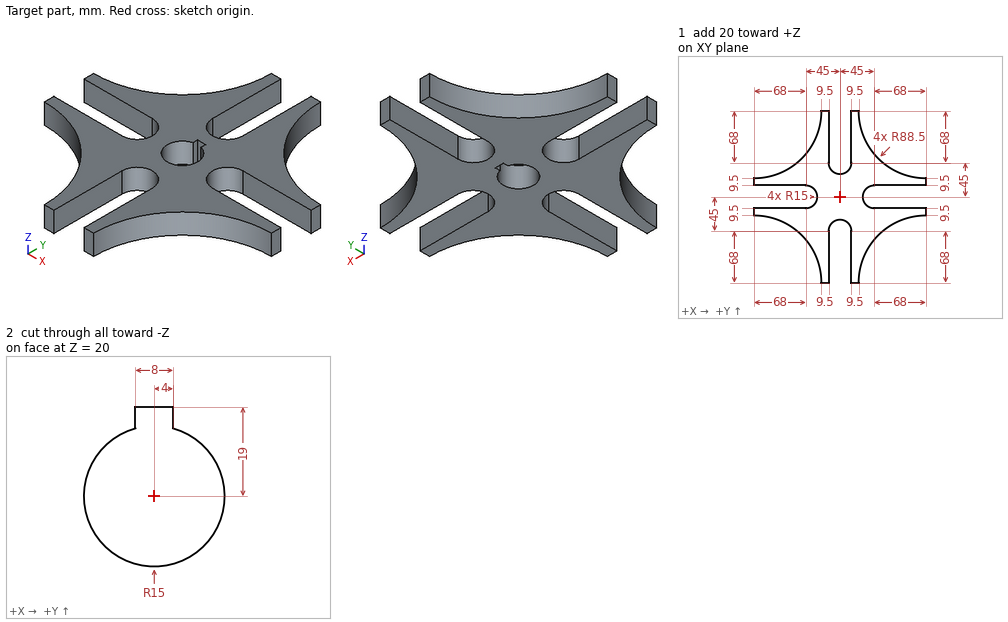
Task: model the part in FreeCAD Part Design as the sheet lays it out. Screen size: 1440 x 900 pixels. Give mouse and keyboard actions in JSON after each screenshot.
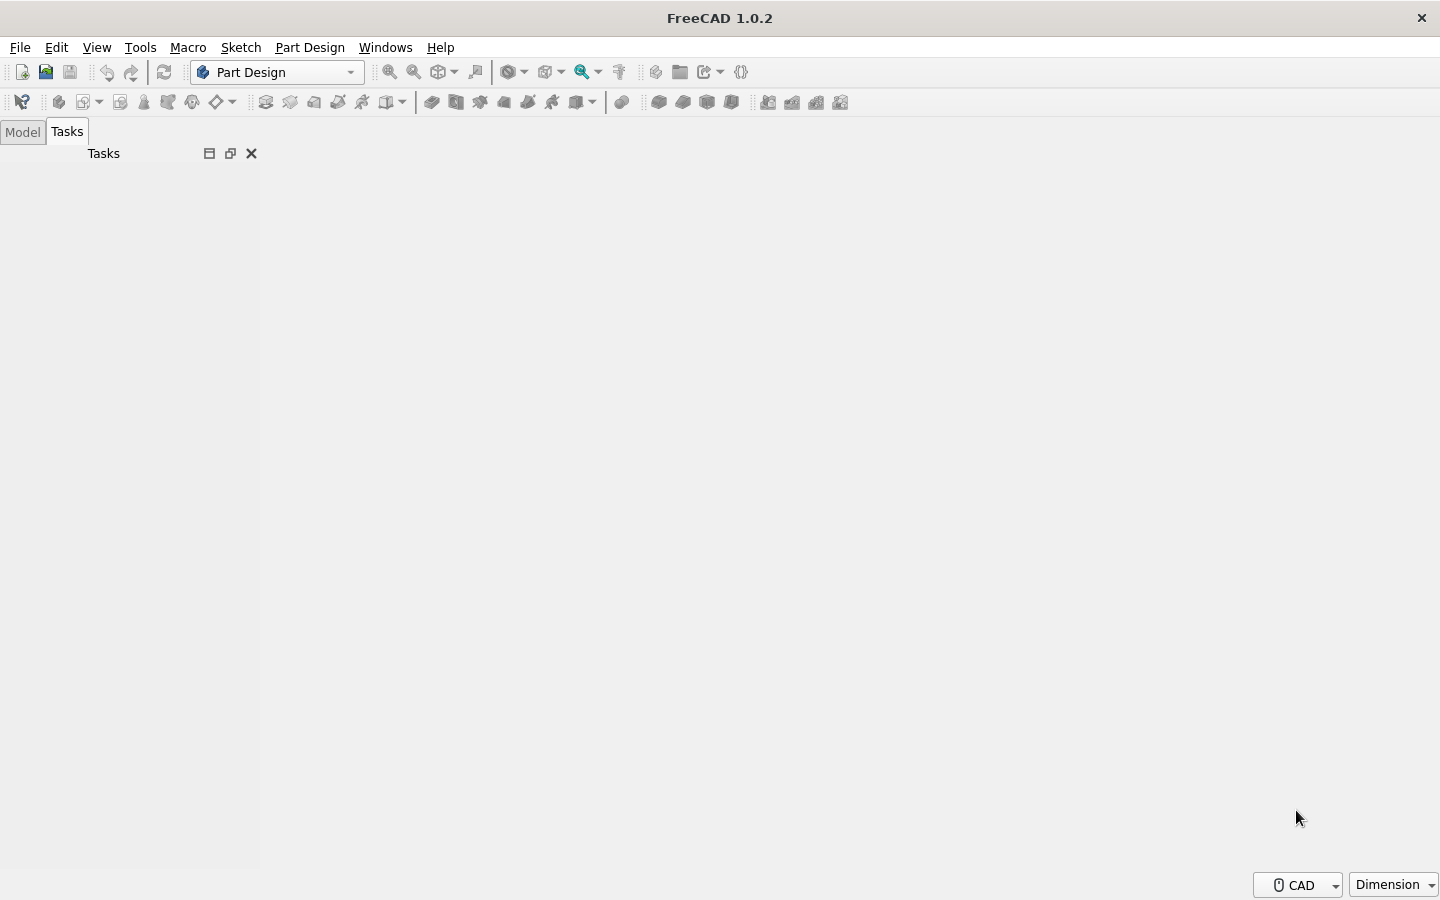
{"action": "left_click", "coordinate": [22, 72]}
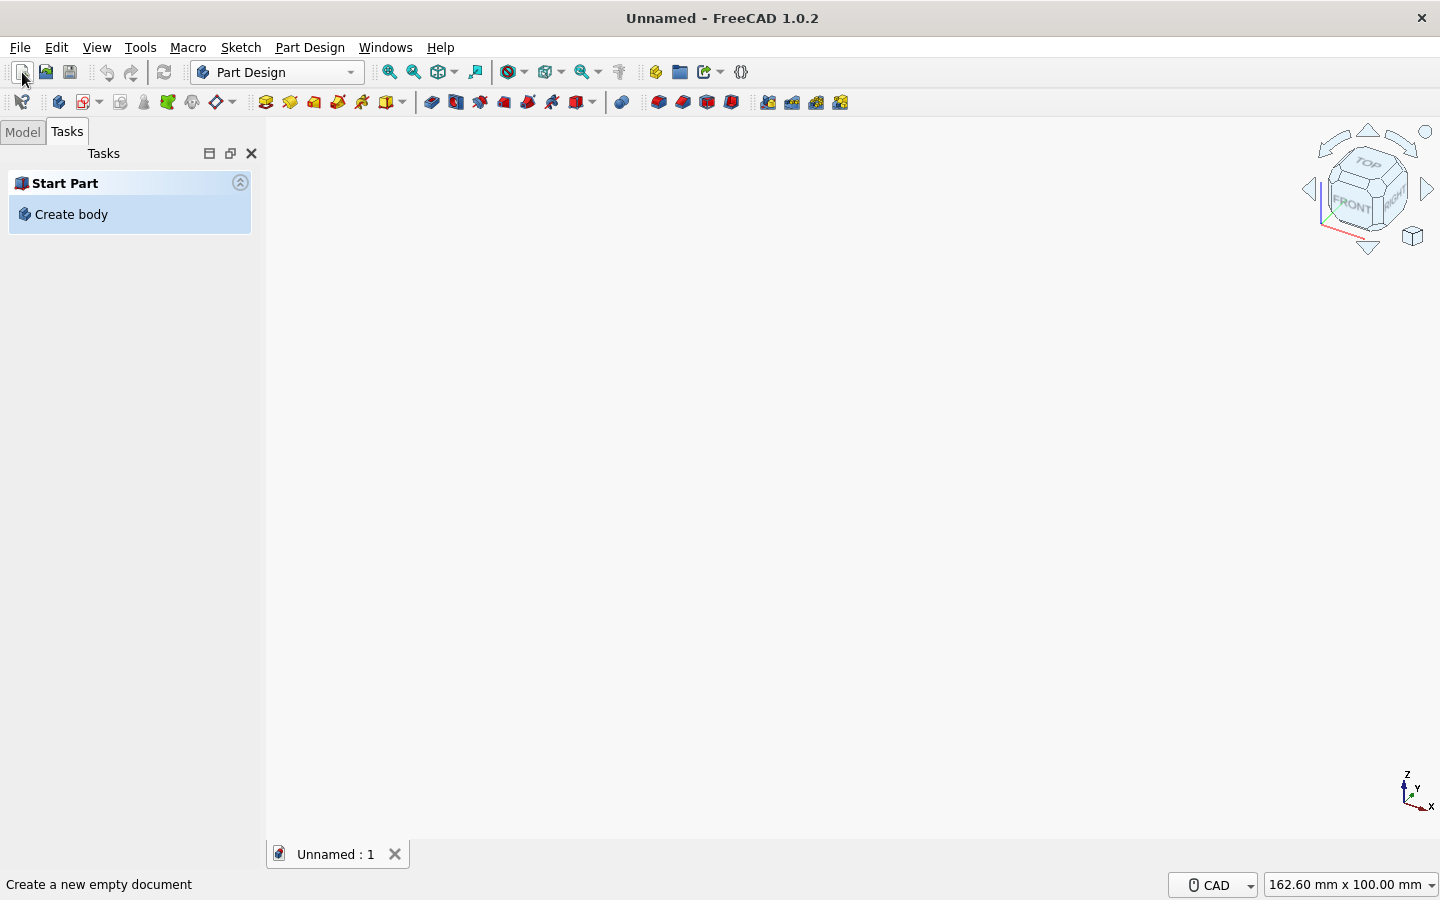
{"action": "left_click", "coordinate": [84, 102]}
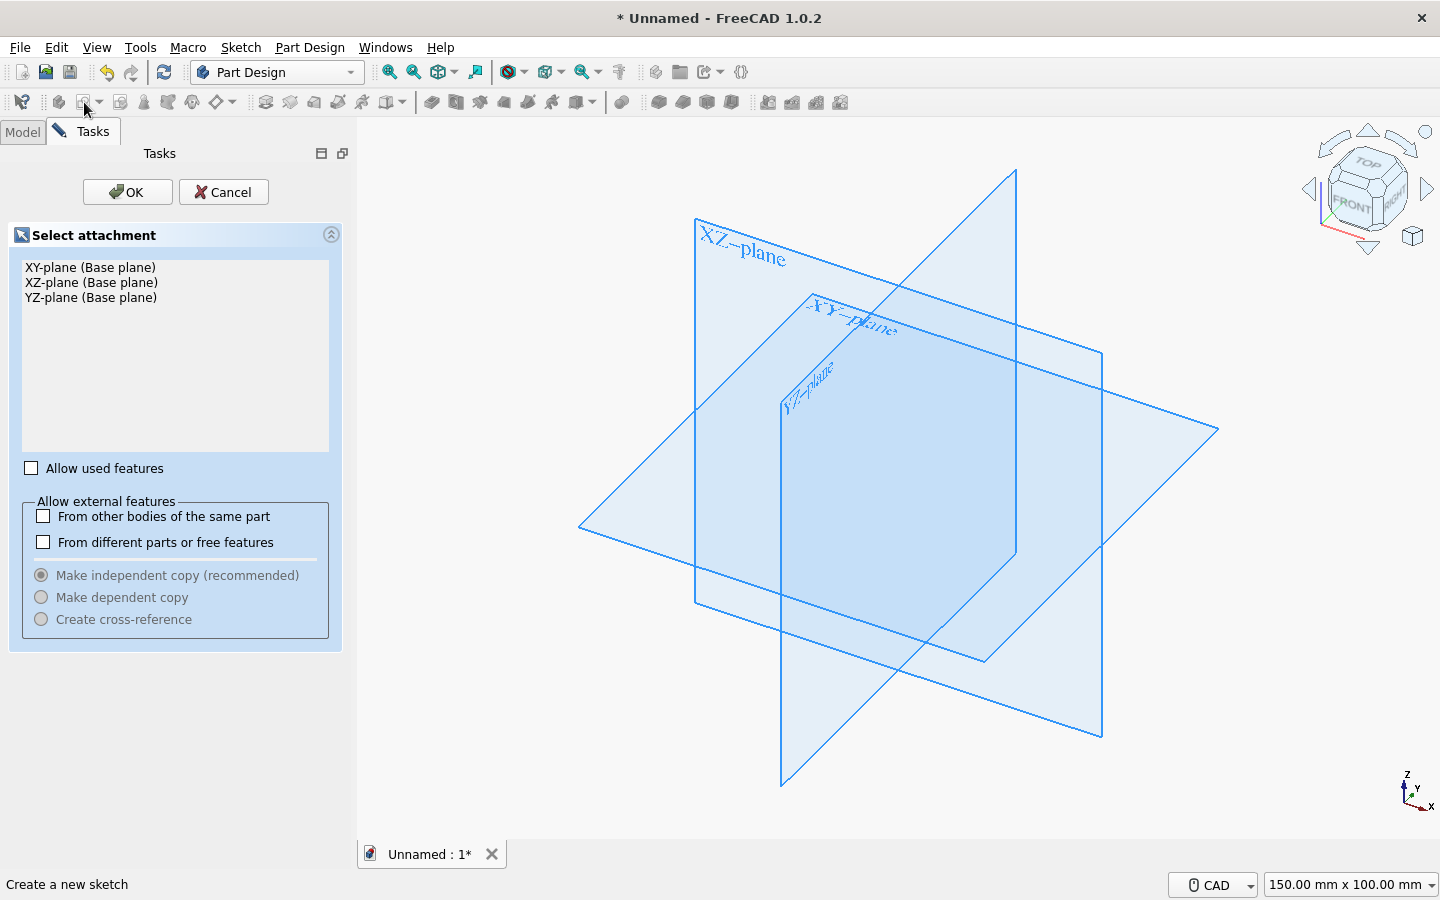
{"action": "left_click", "coordinate": [82, 268]}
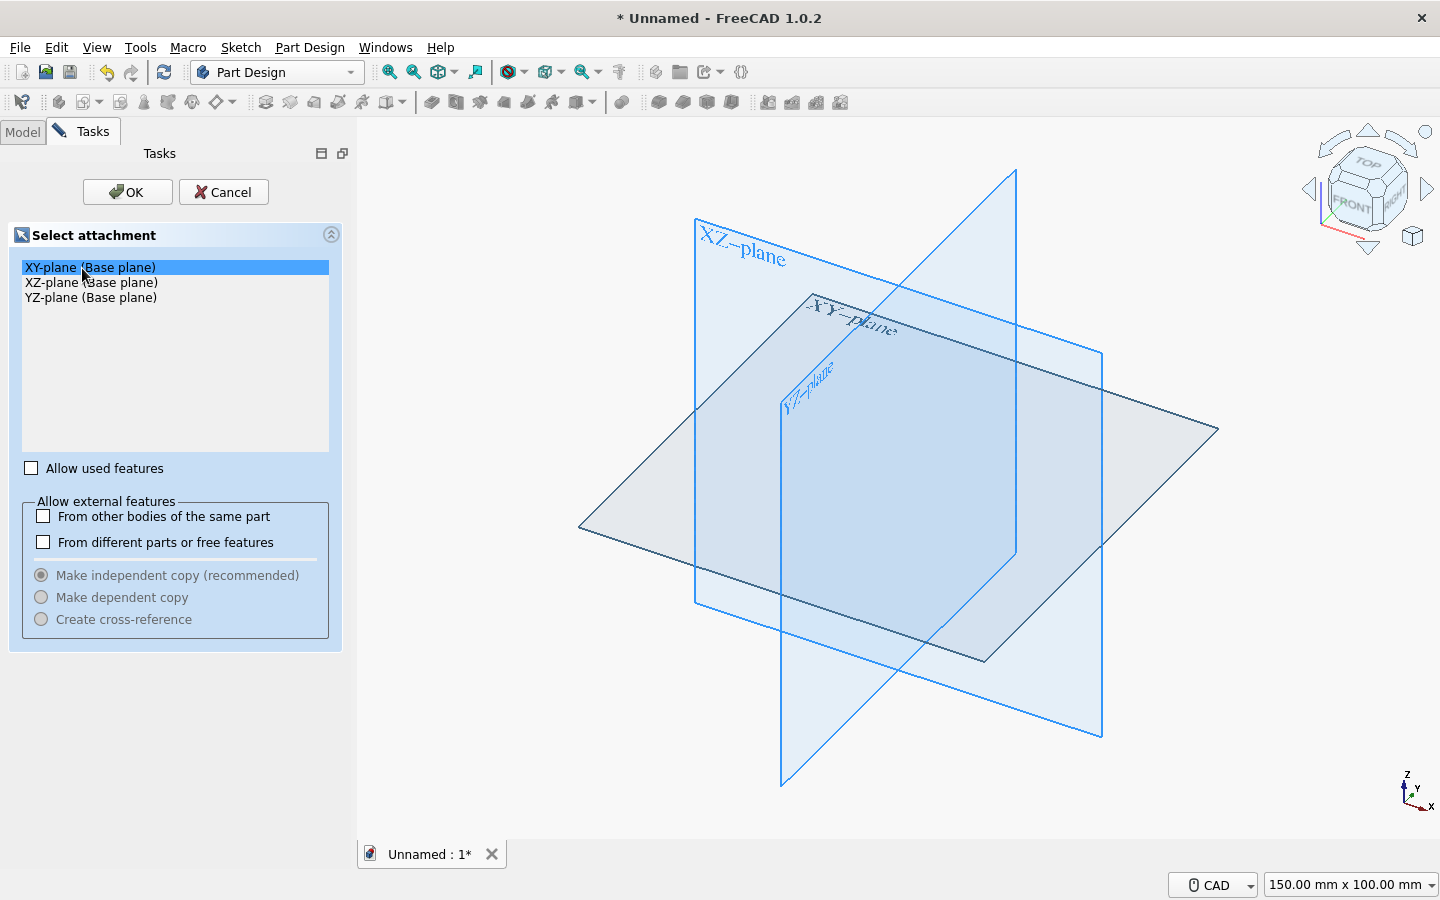
{"action": "left_click", "coordinate": [128, 192]}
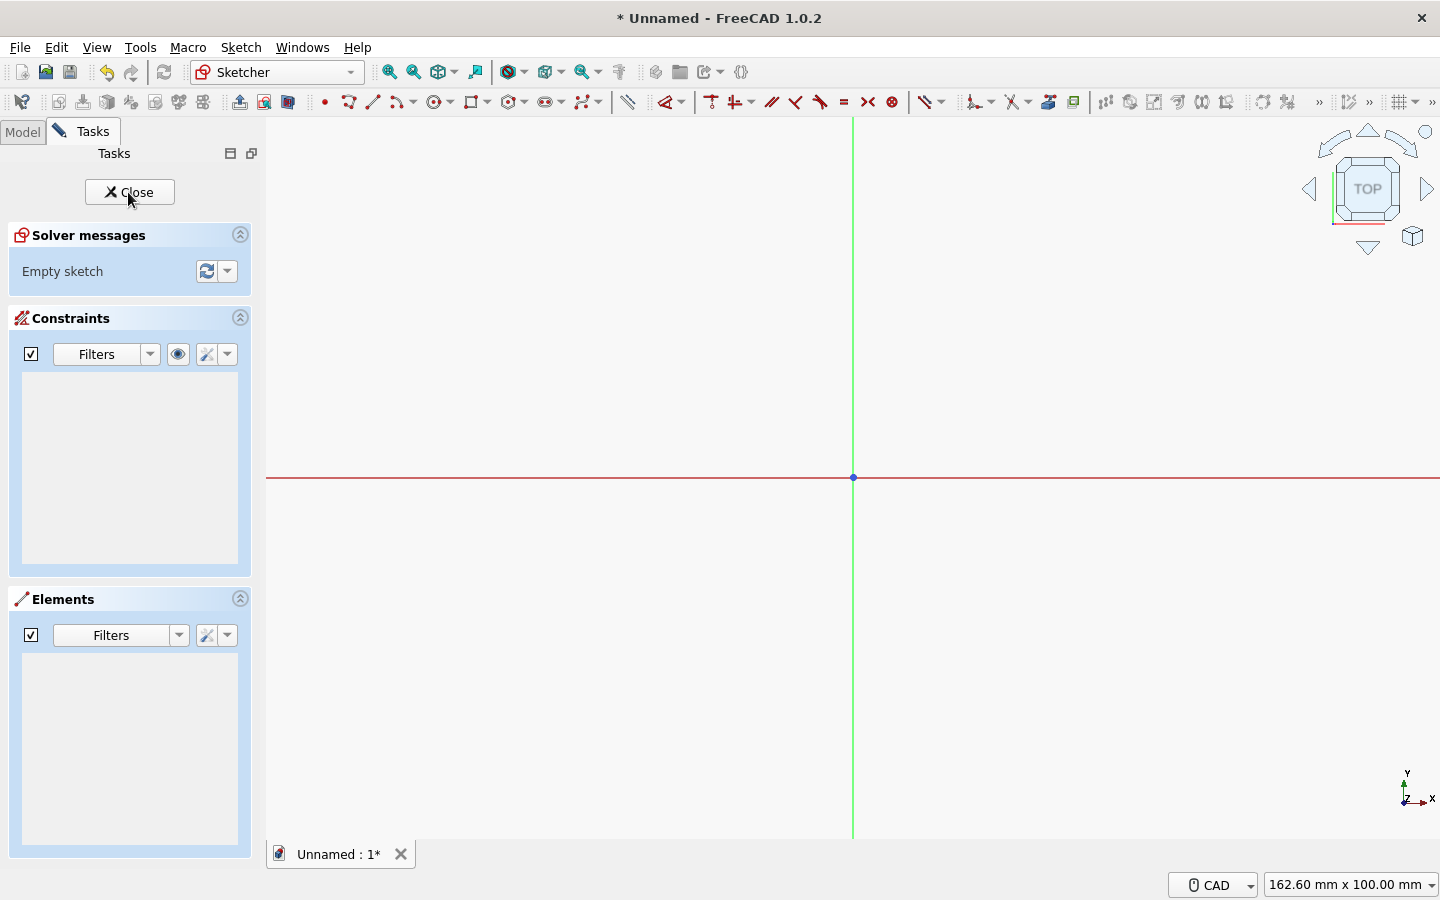
{"action": "scroll", "coordinate": [755, 478], "scroll_direction": "down", "scroll_amount": 6}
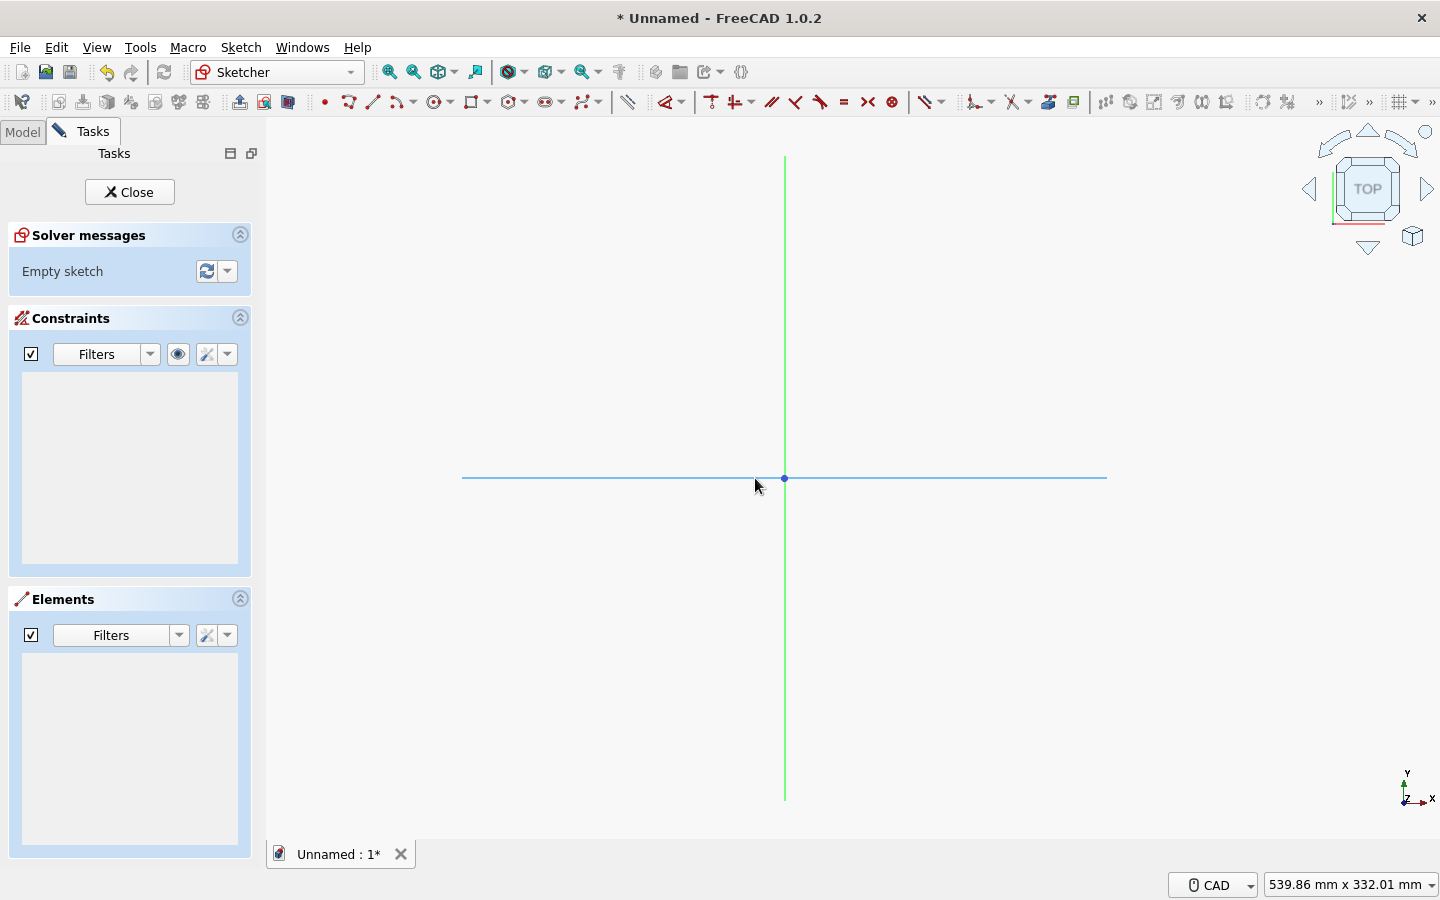
{"action": "left_click", "coordinate": [350, 102]}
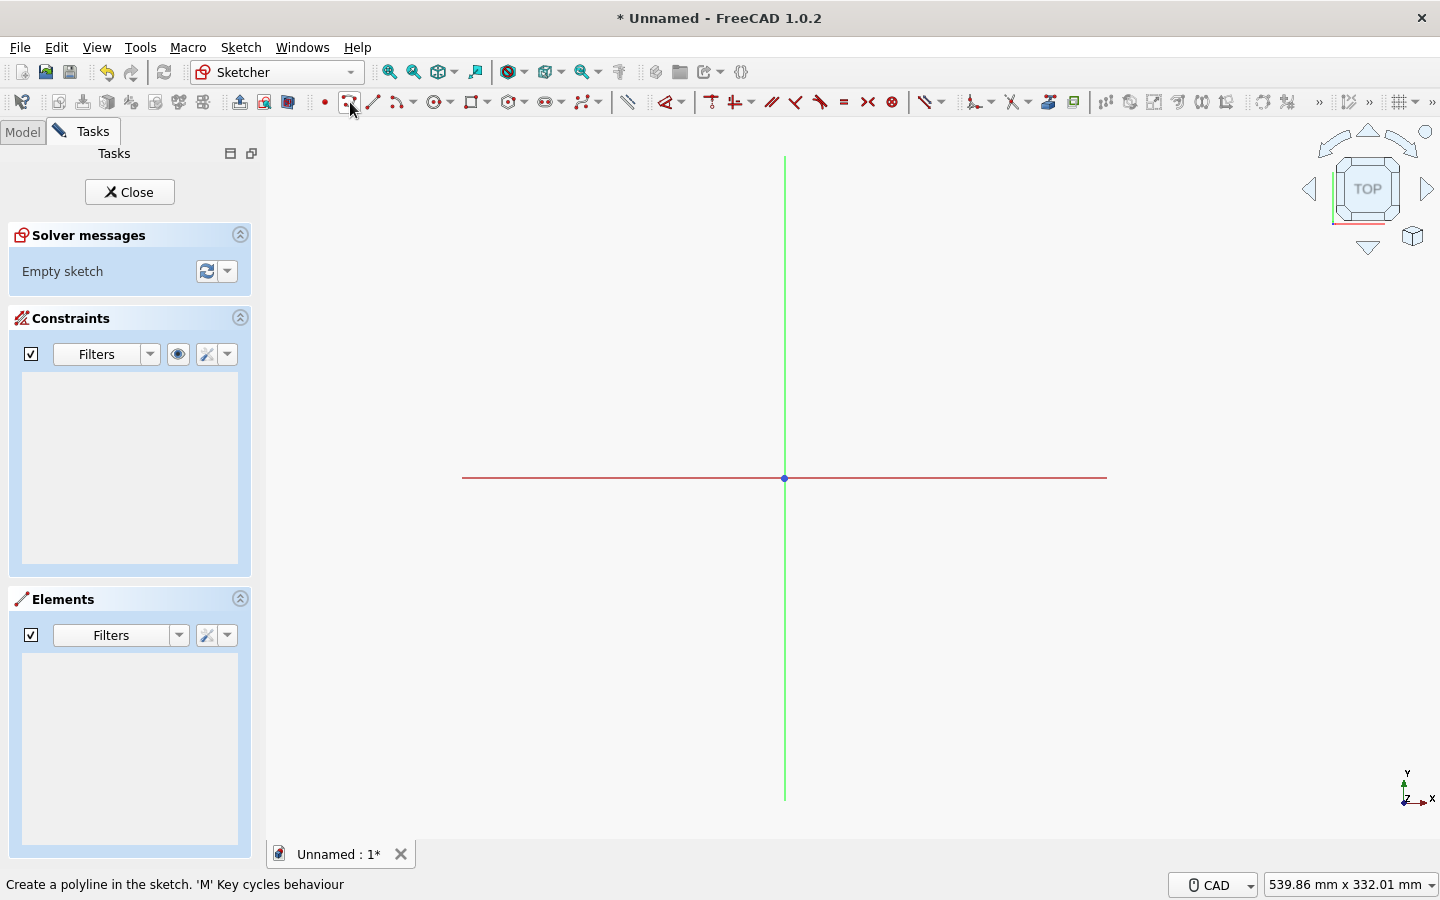
{"action": "left_click", "coordinate": [883, 446]}
{"action": "left_click", "coordinate": [1031, 446]}
{"action": "left_click", "coordinate": [1031, 425]}
{"action": "right_click", "coordinate": [1031, 425]}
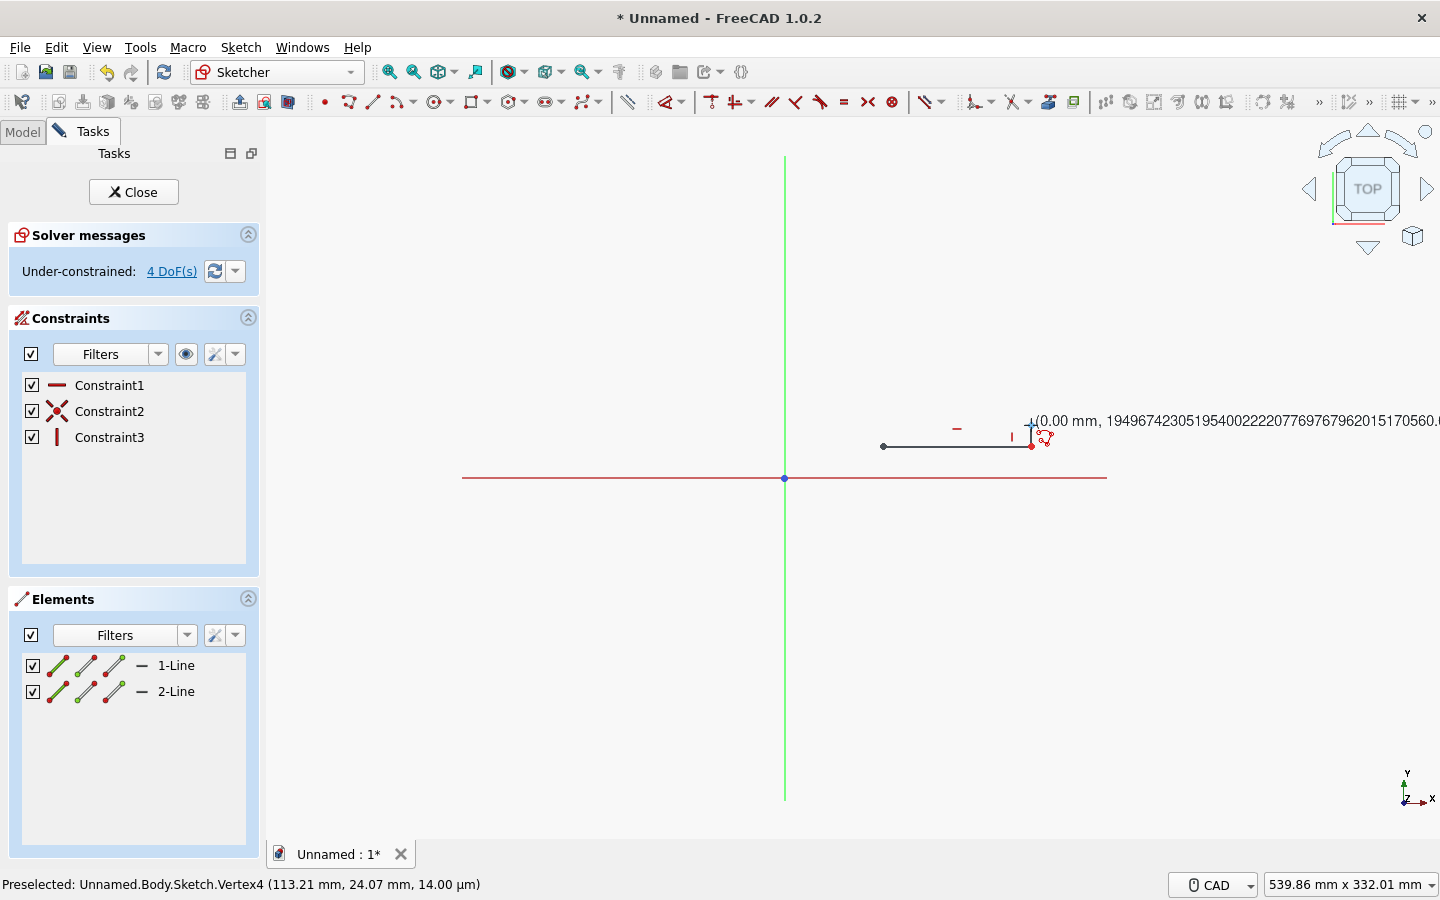
{"action": "left_click", "coordinate": [838, 233]}
{"action": "left_click", "coordinate": [817, 233]}
{"action": "left_click", "coordinate": [817, 380]}
{"action": "right_click", "coordinate": [817, 380]}